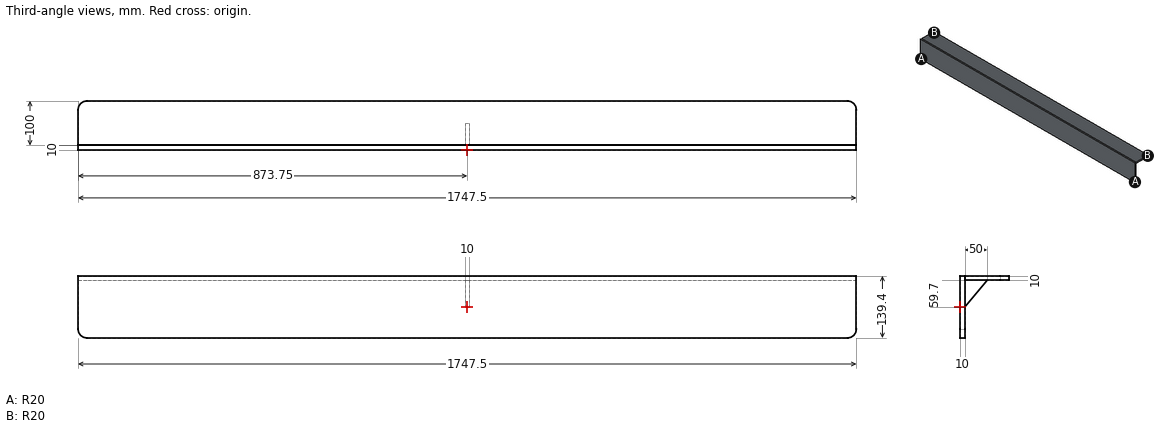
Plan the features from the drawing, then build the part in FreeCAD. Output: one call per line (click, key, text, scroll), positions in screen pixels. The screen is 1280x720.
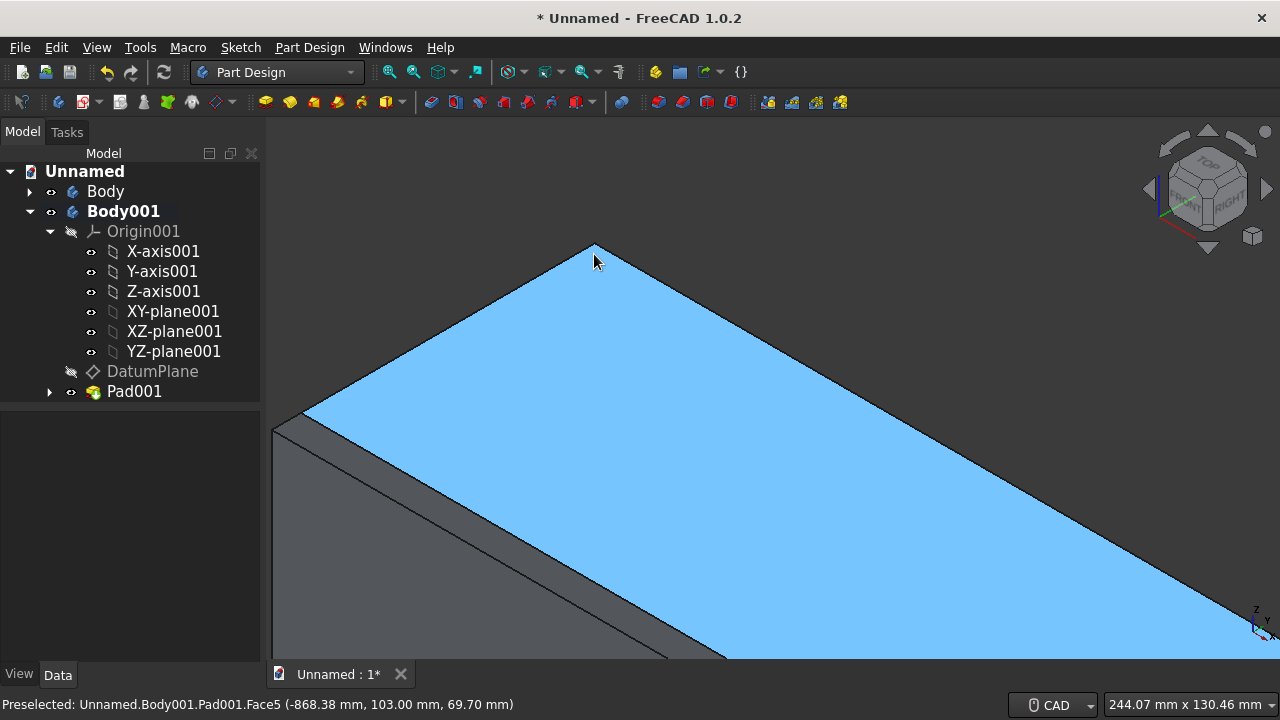
click(390, 72)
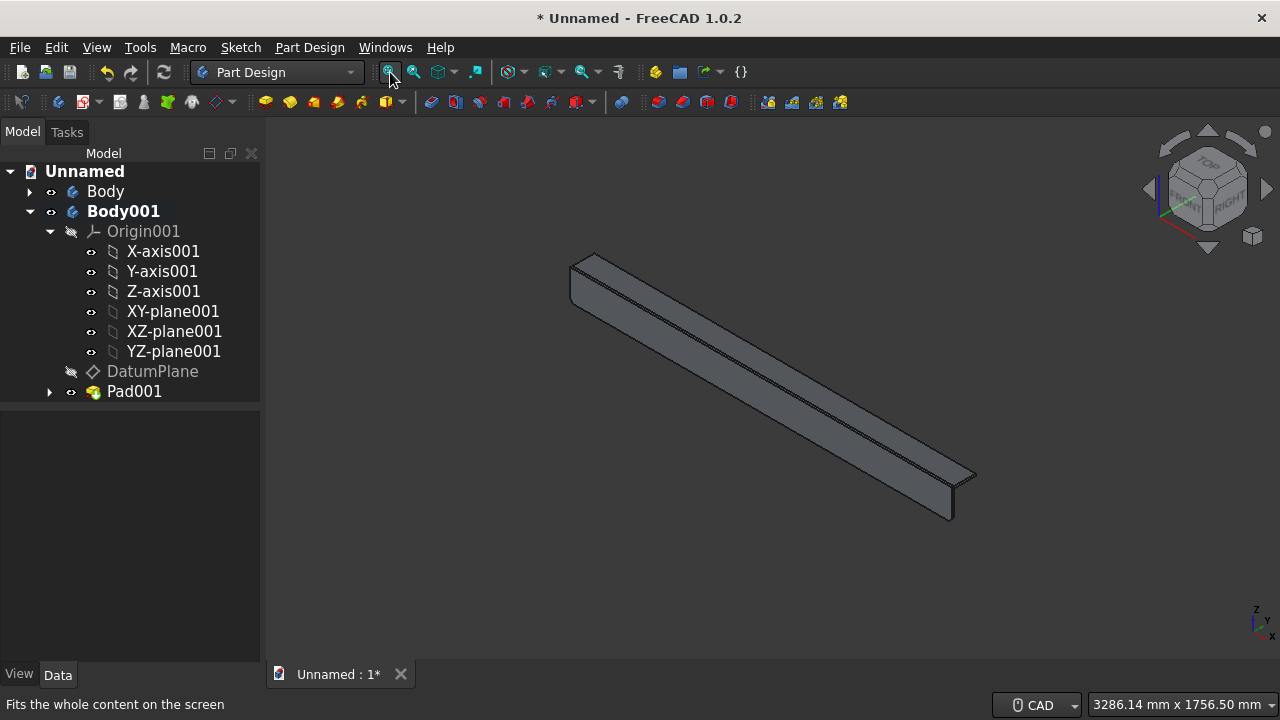
key(2)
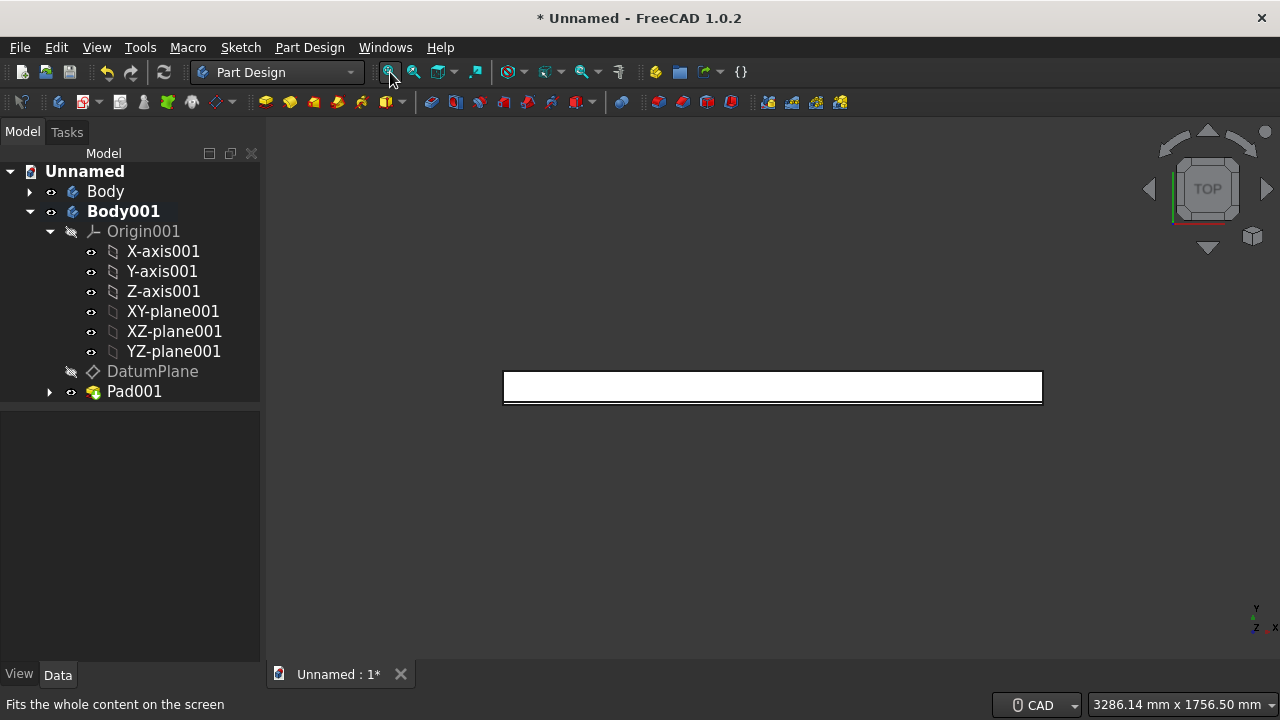
scroll(503, 370, up, 13)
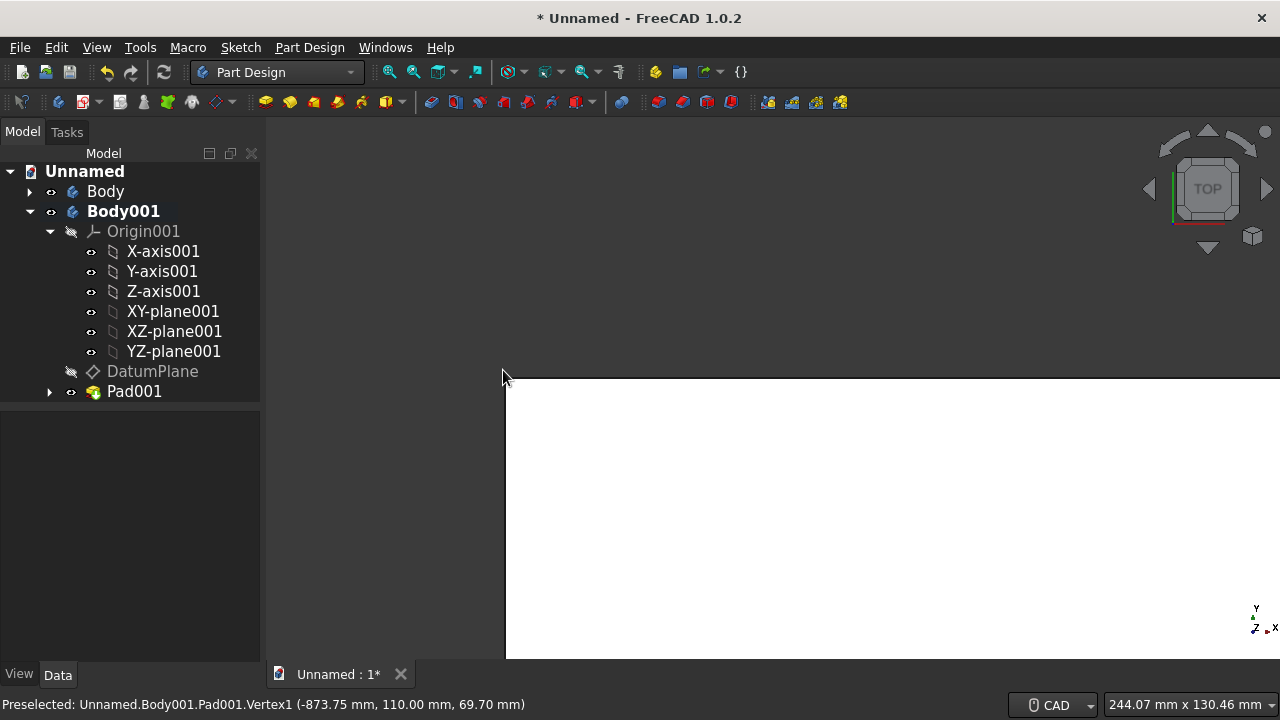
click(390, 72)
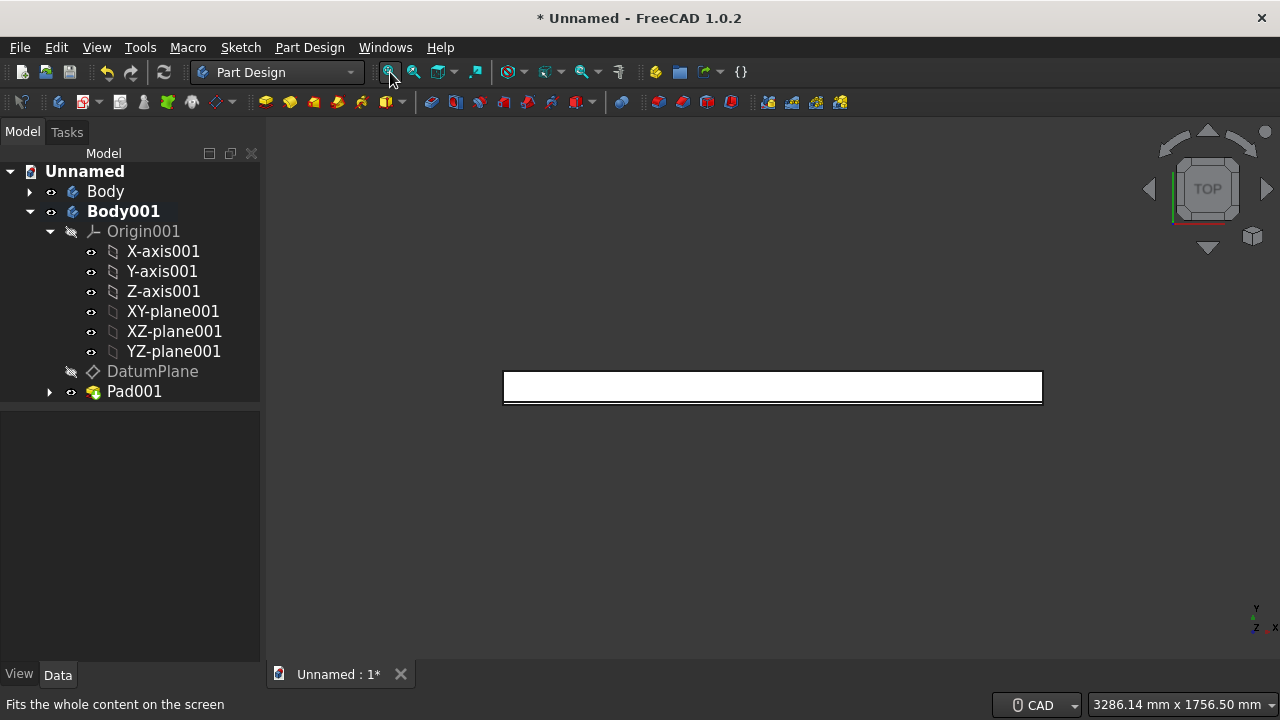
key(1)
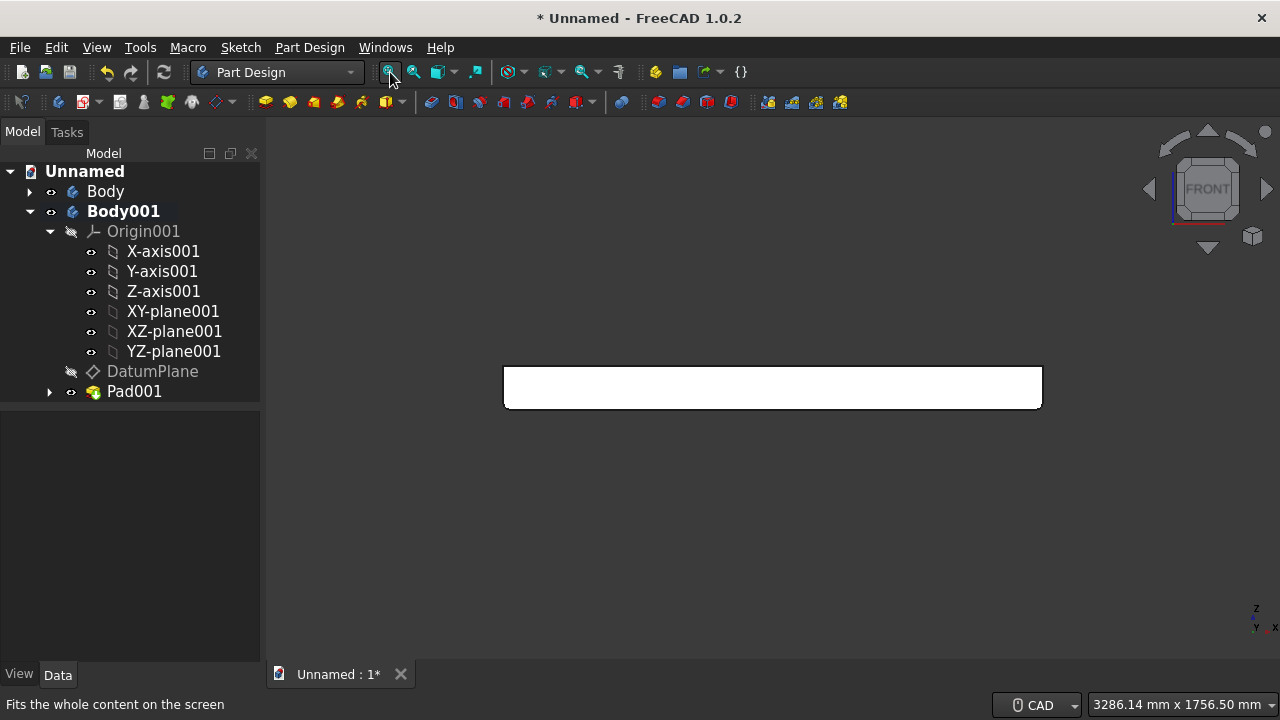
scroll(503, 367, up, 13)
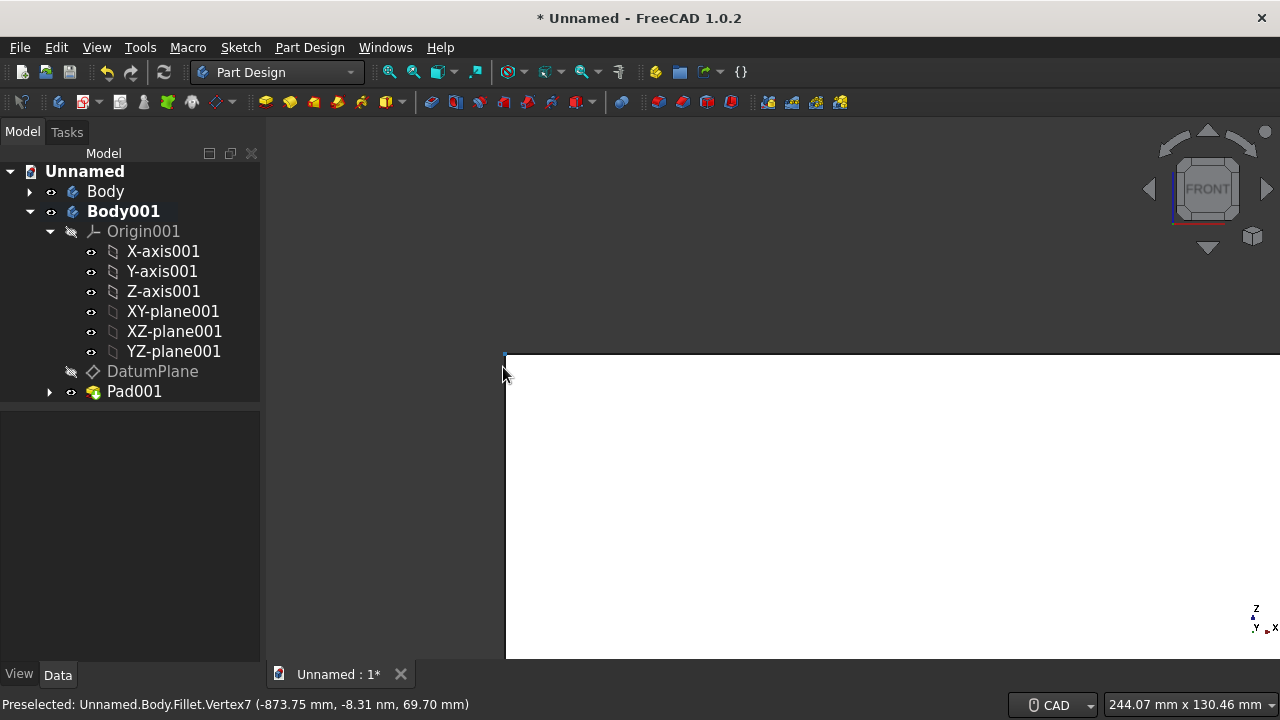
click(390, 72)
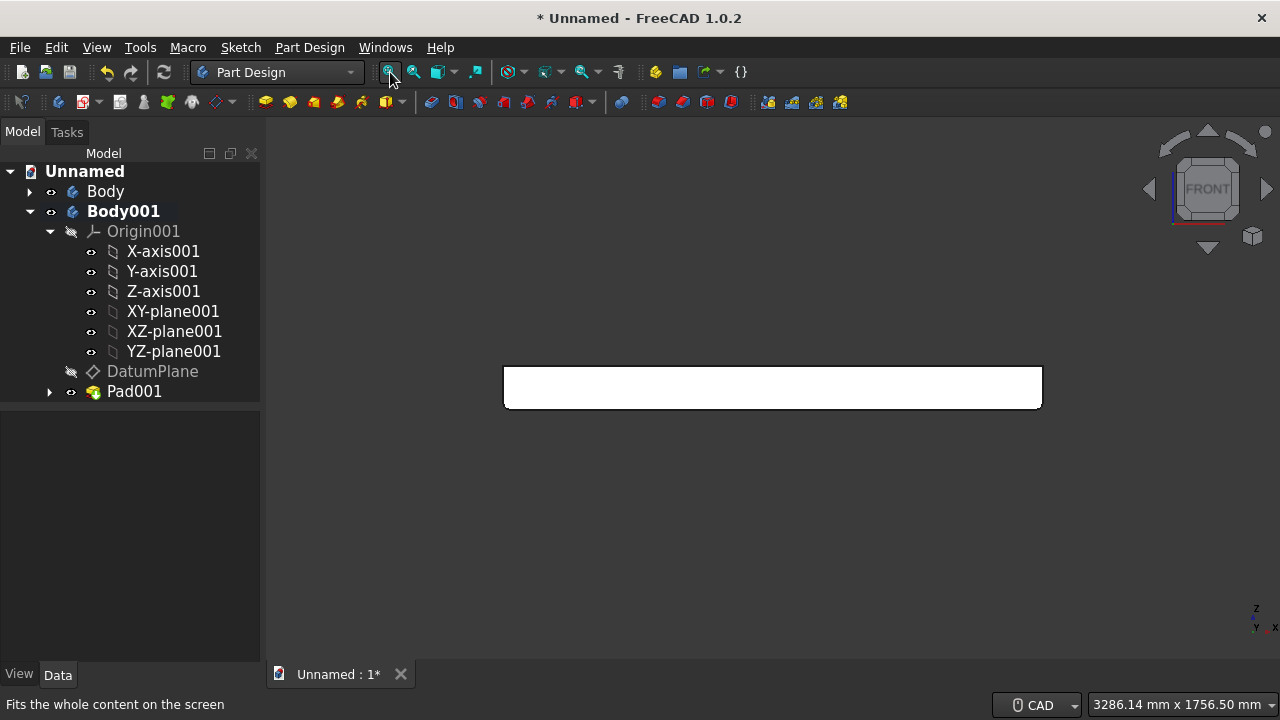
key(3)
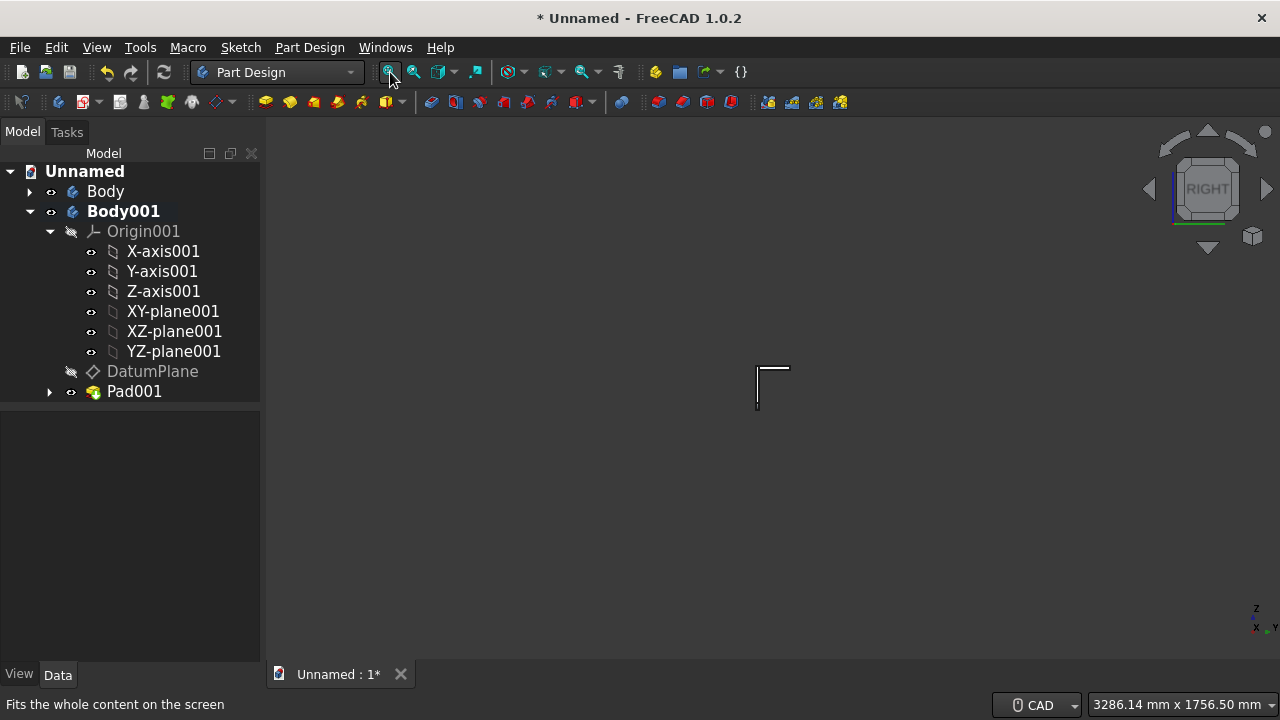
click(390, 72)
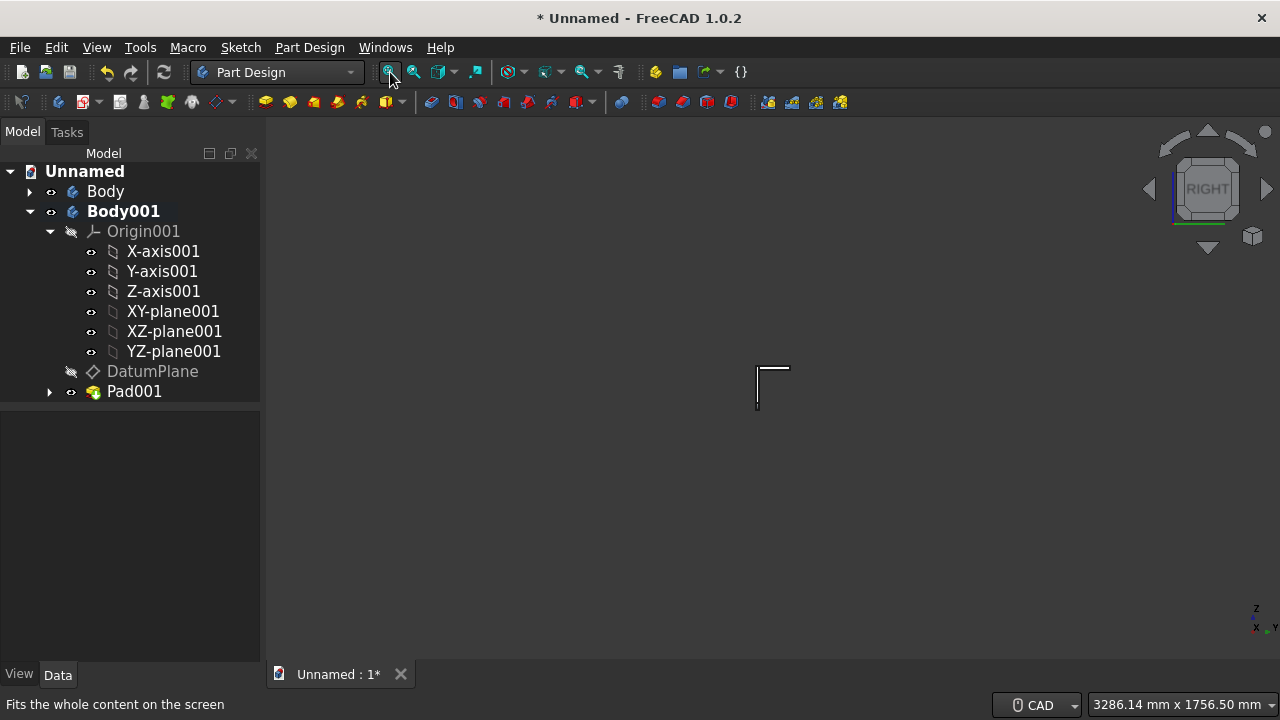
scroll(790, 367, up, 13)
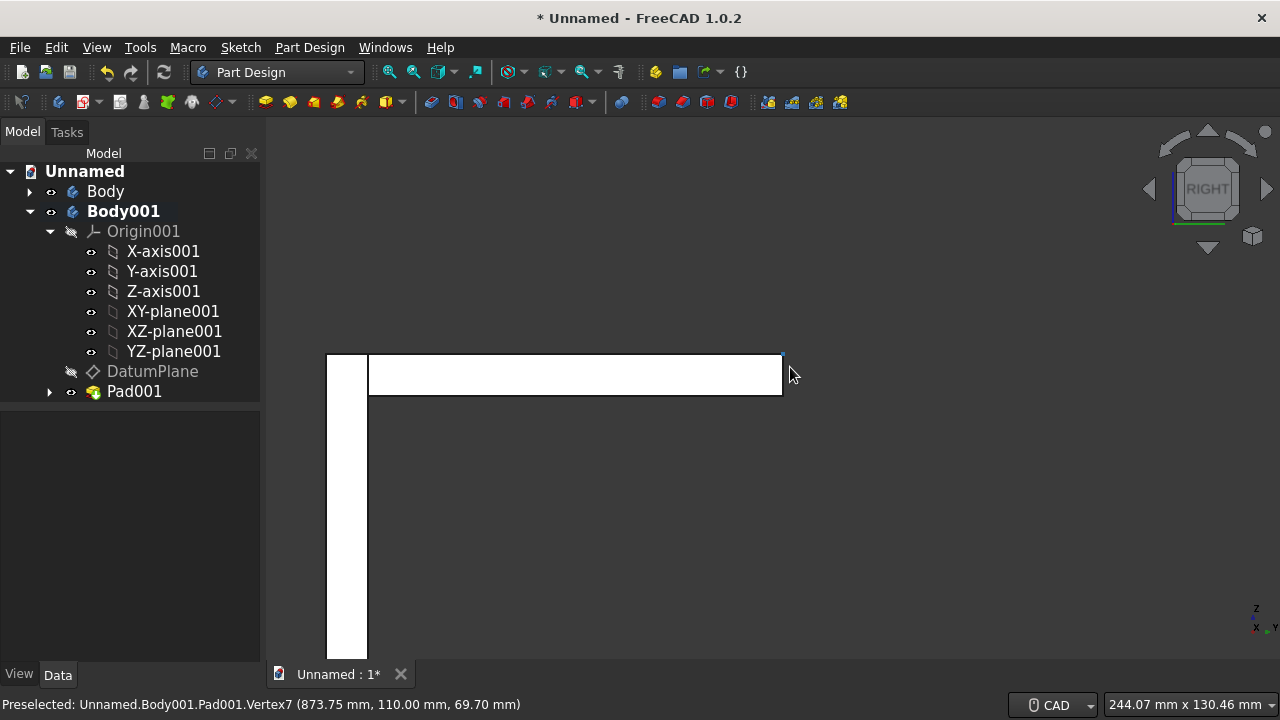
click(783, 374)